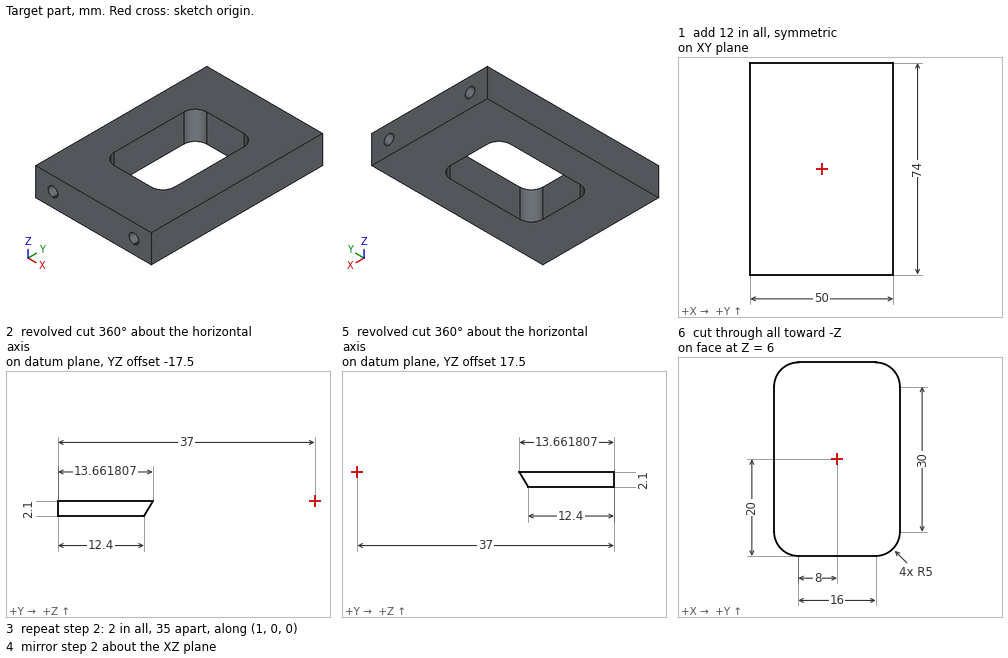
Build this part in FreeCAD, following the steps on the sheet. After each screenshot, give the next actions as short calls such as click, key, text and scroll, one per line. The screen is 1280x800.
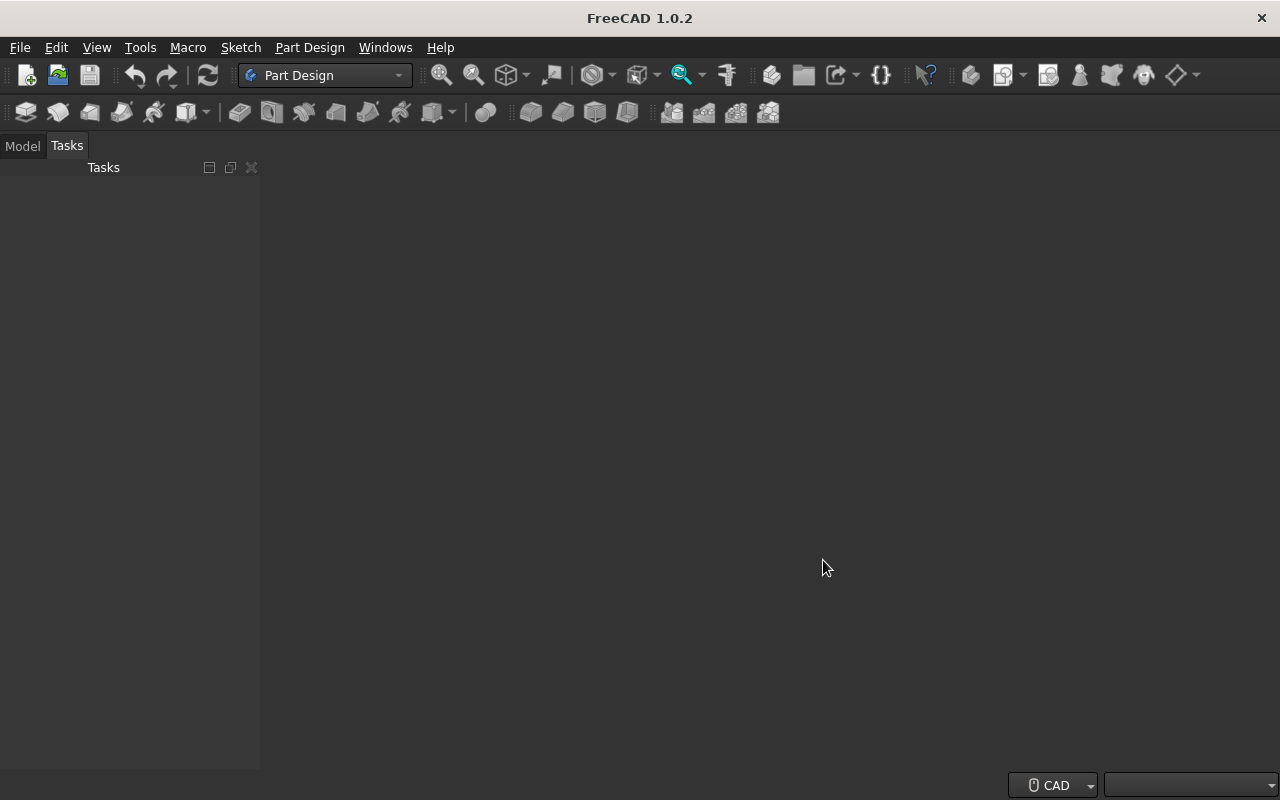
click(26, 76)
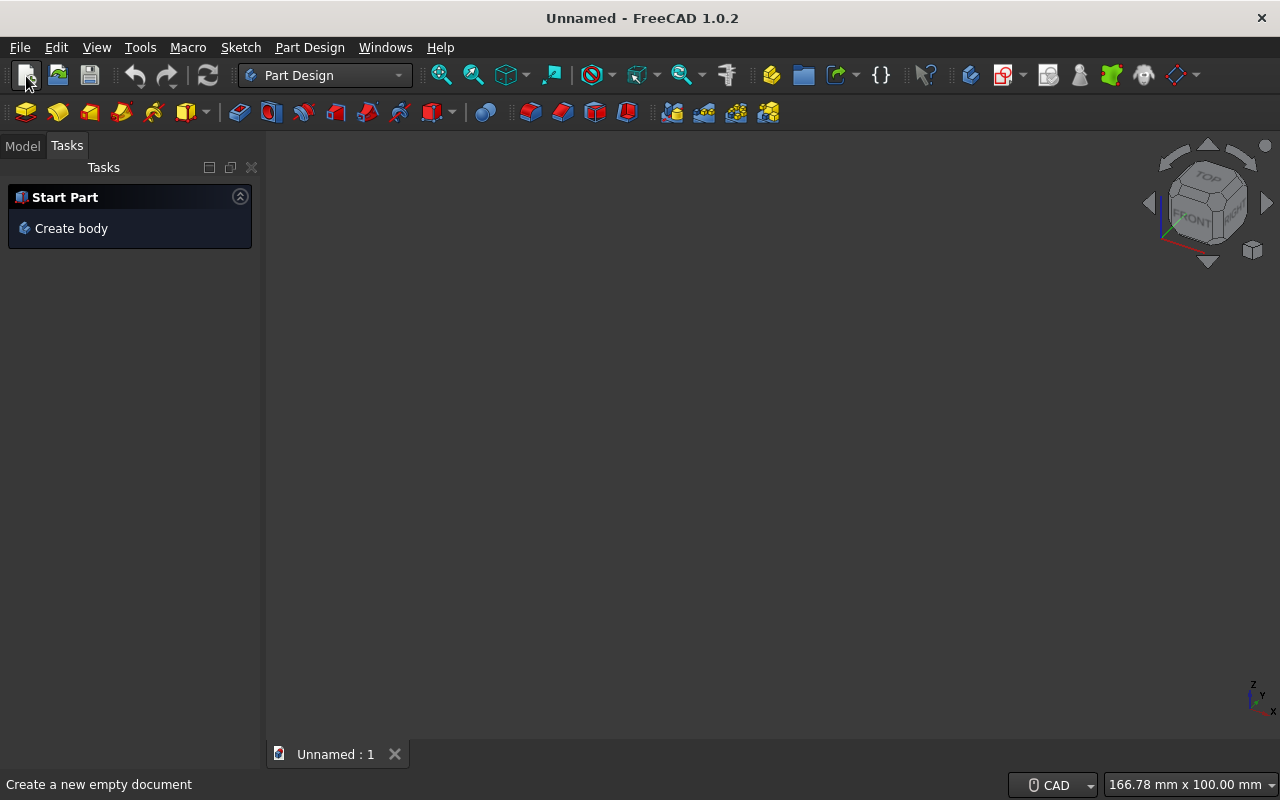
click(1004, 76)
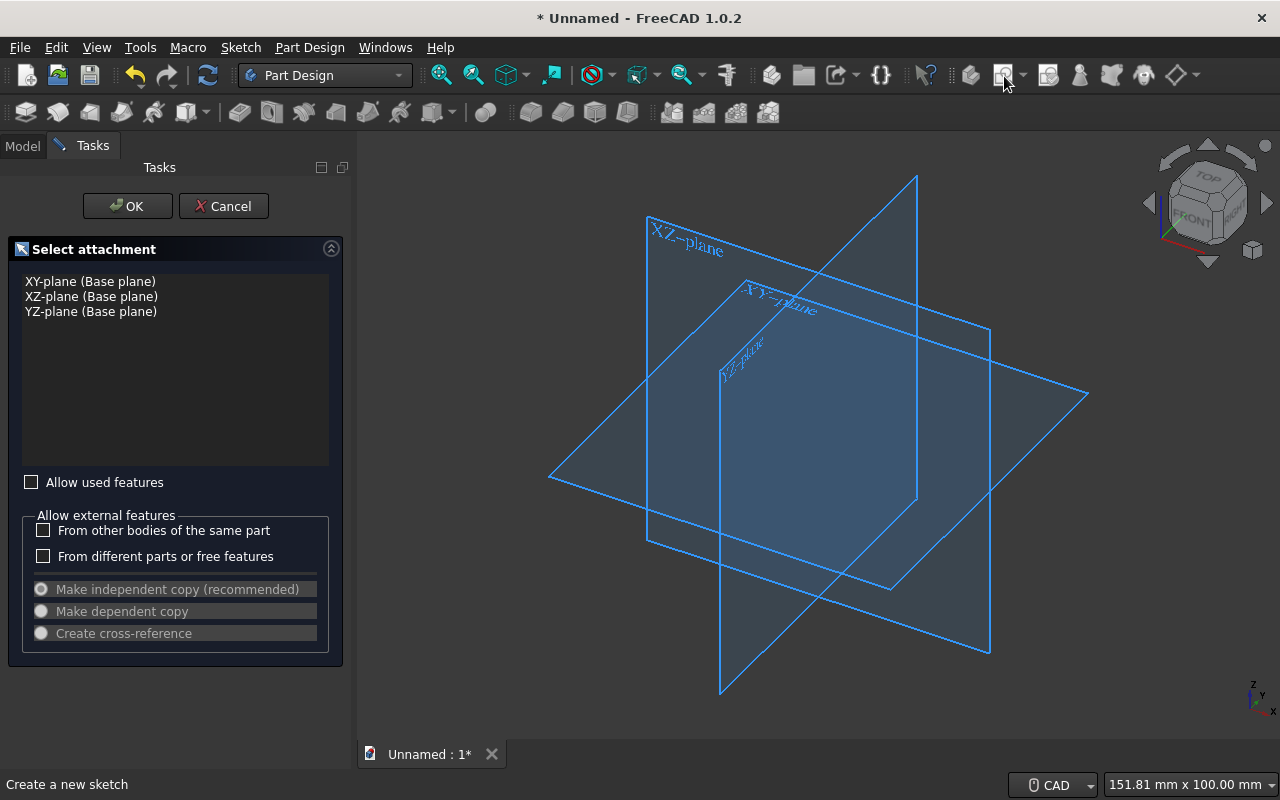
click(82, 282)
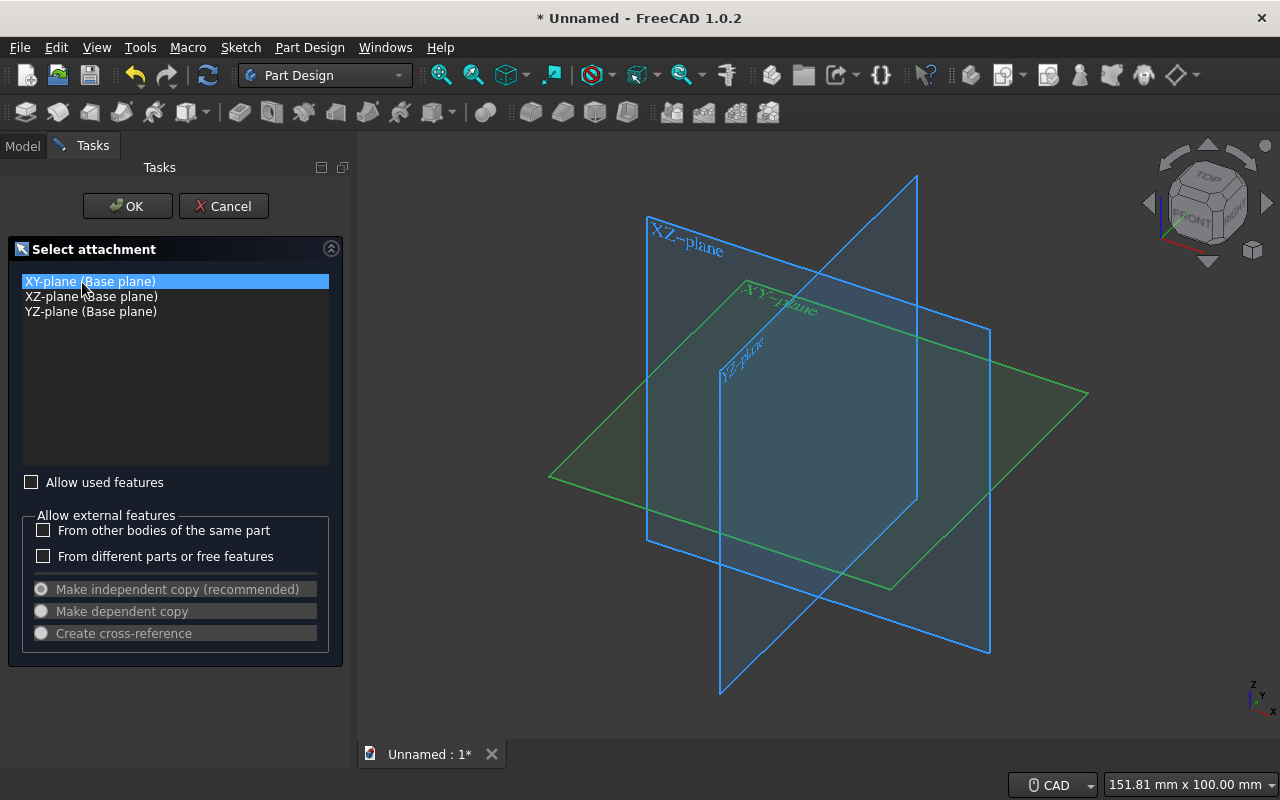
click(128, 206)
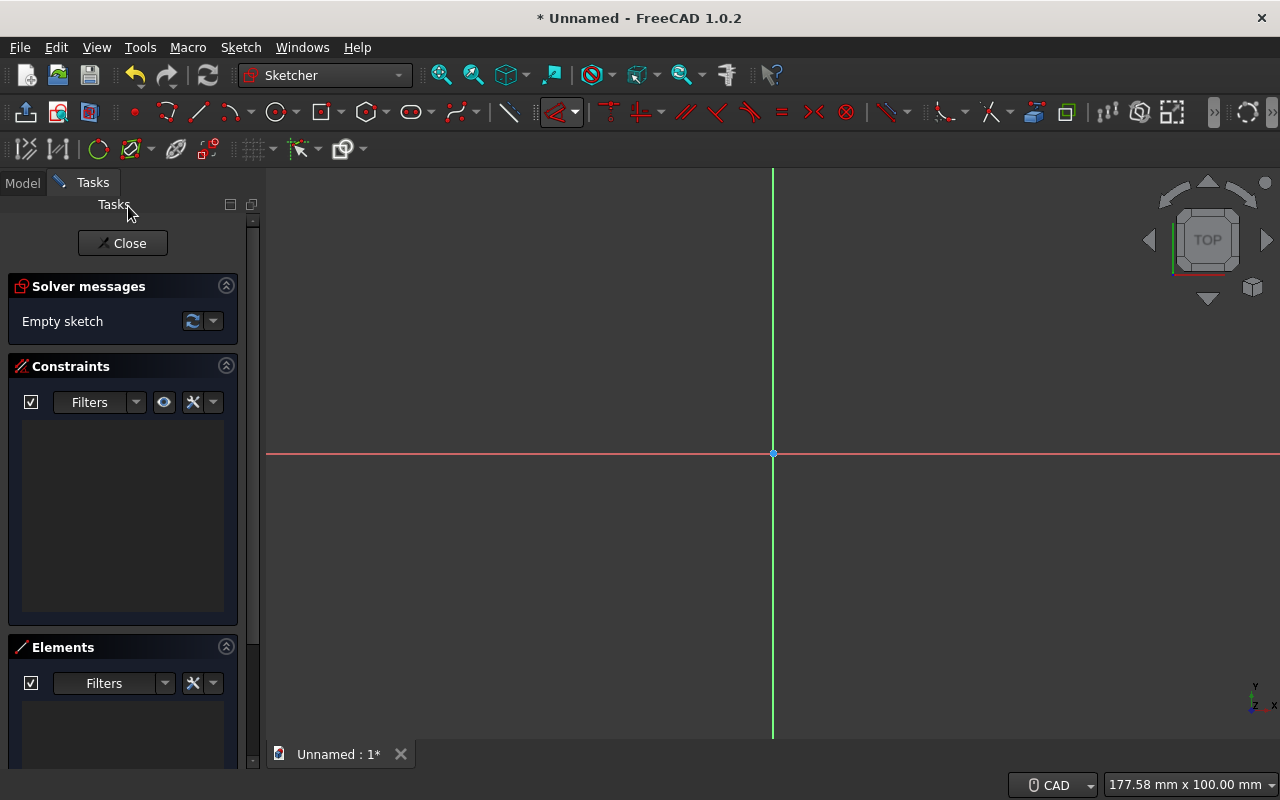
click(322, 112)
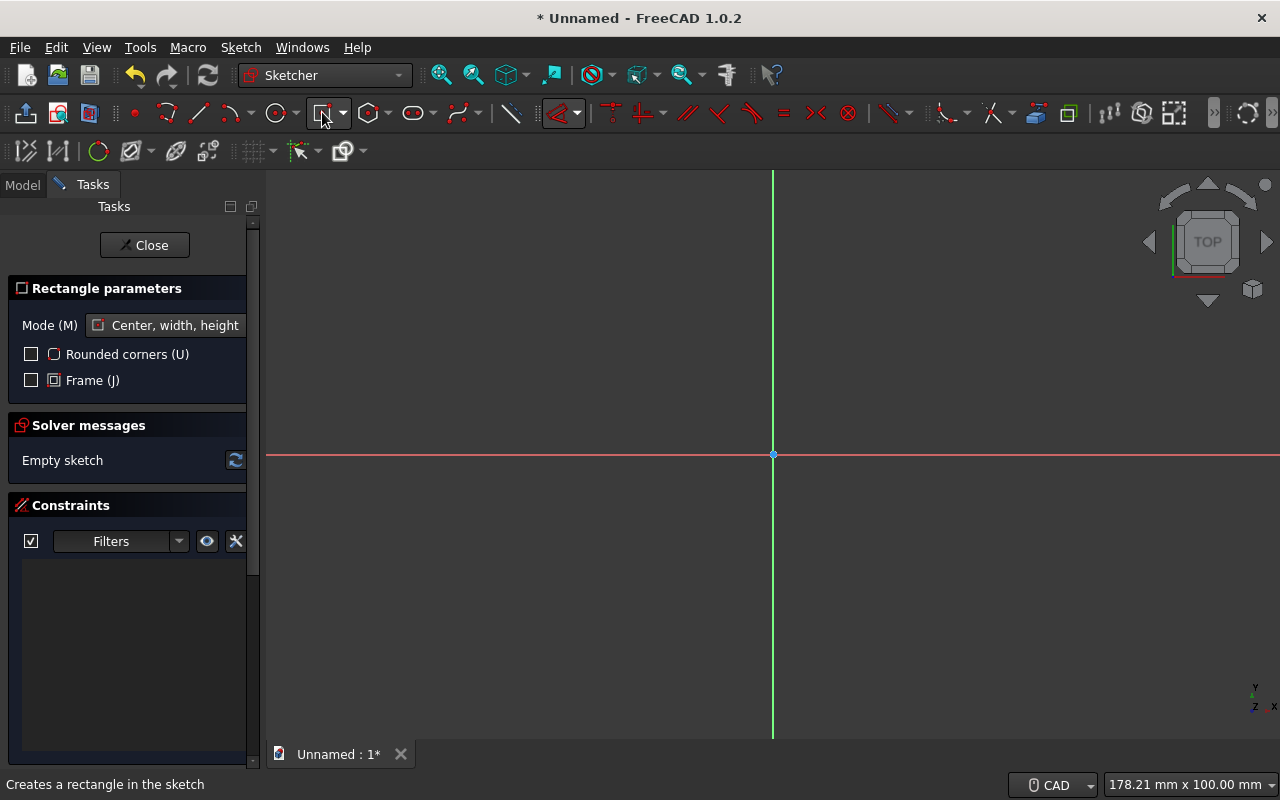
click(773, 454)
click(915, 244)
key(Escape)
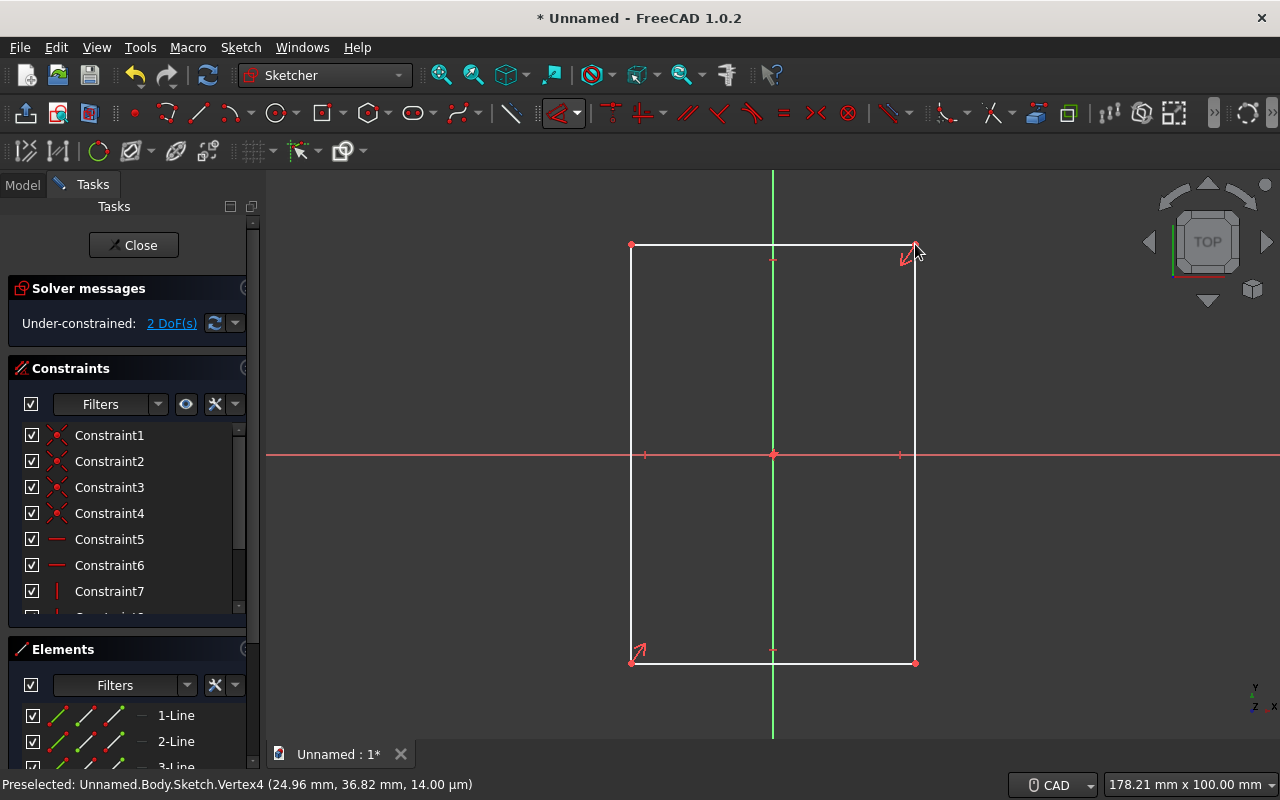
click(716, 664)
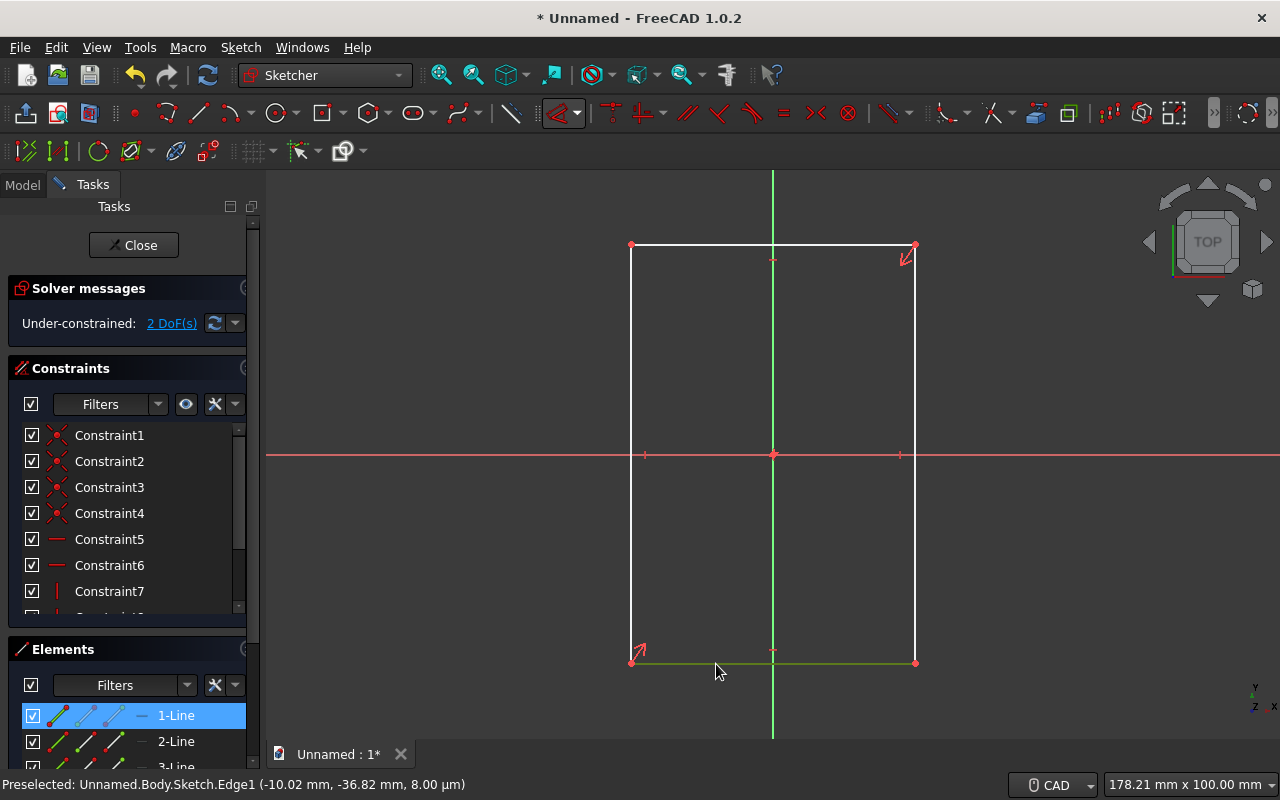
key(l)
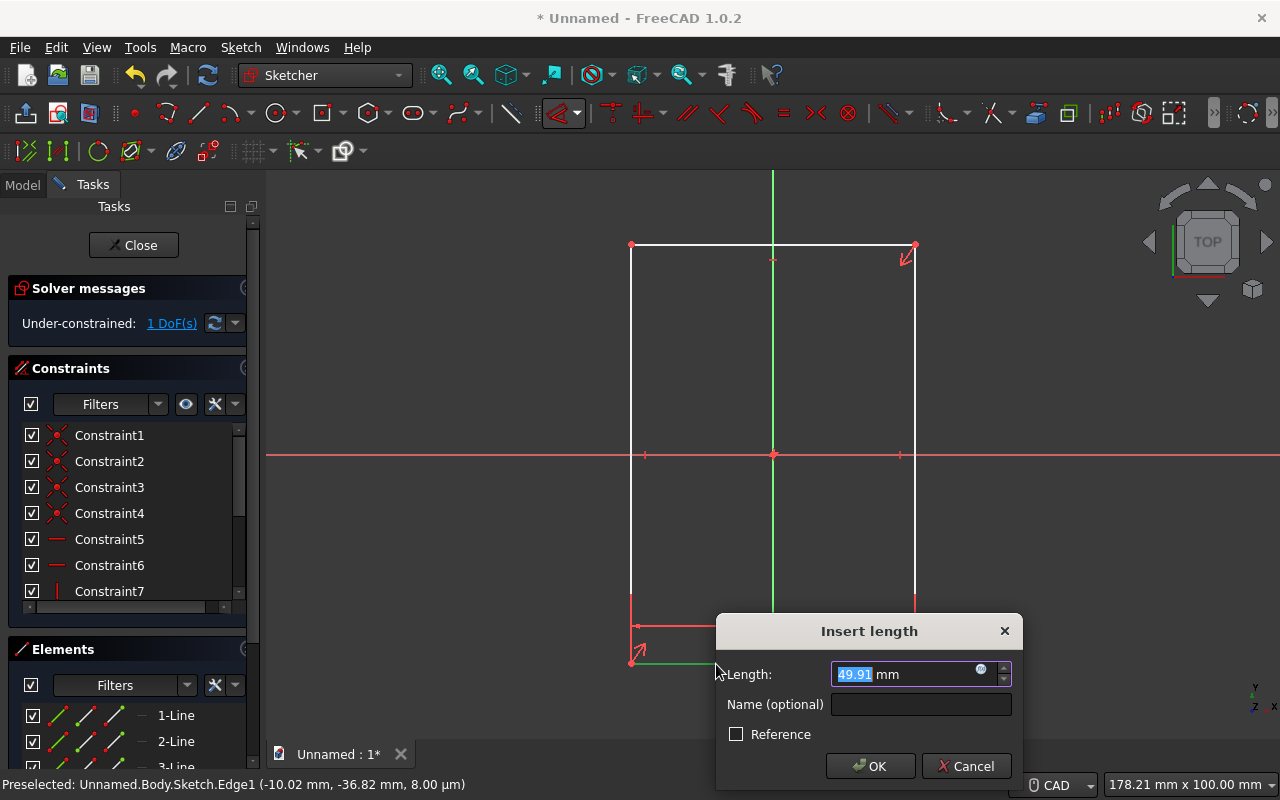
text(50)
key(Return)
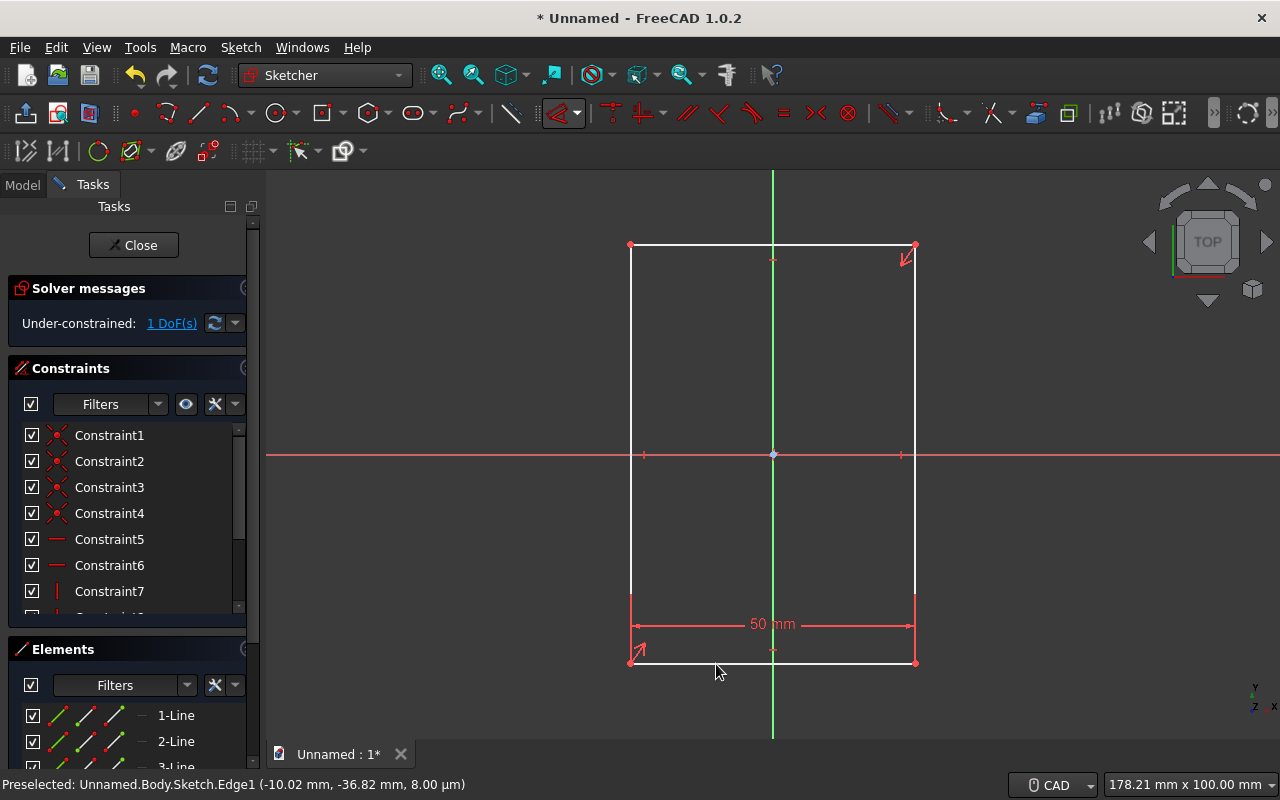
click(915, 538)